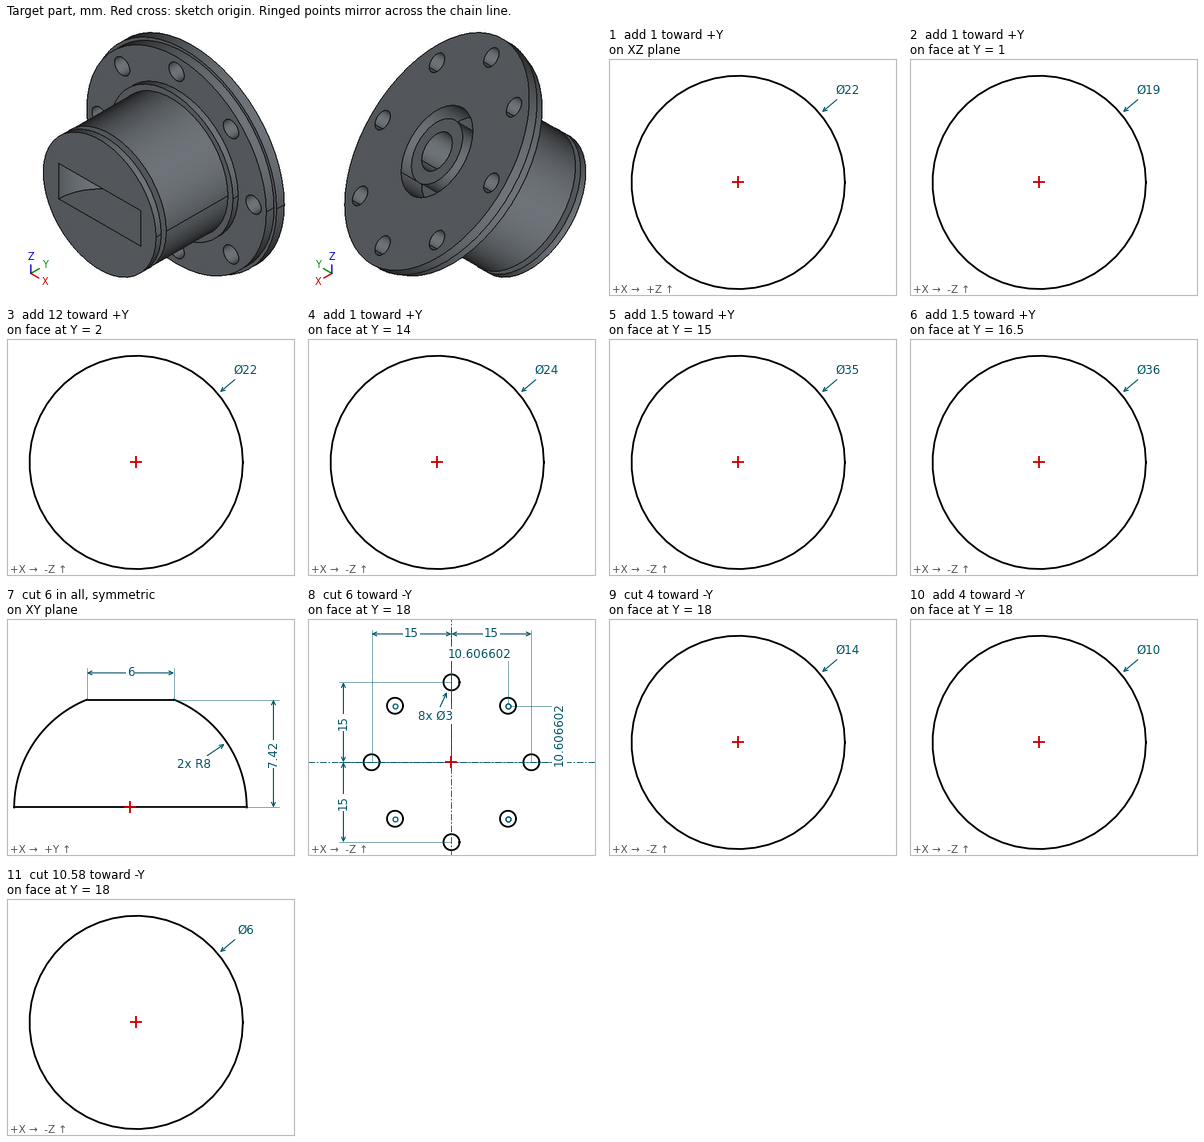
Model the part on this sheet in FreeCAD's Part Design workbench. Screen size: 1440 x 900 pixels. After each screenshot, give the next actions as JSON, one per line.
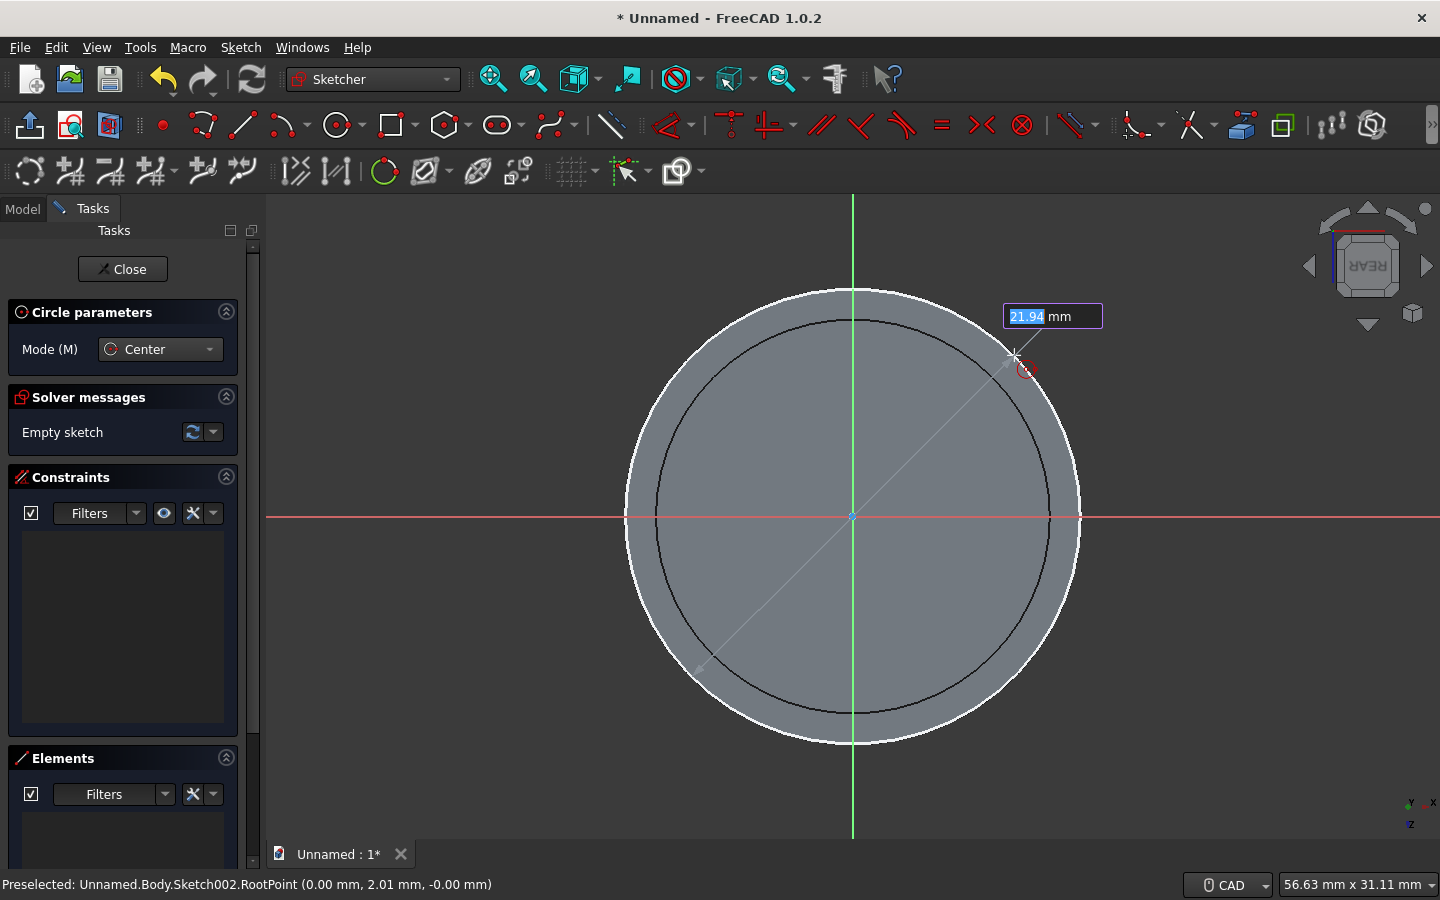
{"action": "type", "text": "22"}
{"action": "key", "text": "Return"}
{"action": "key", "text": "Escape"}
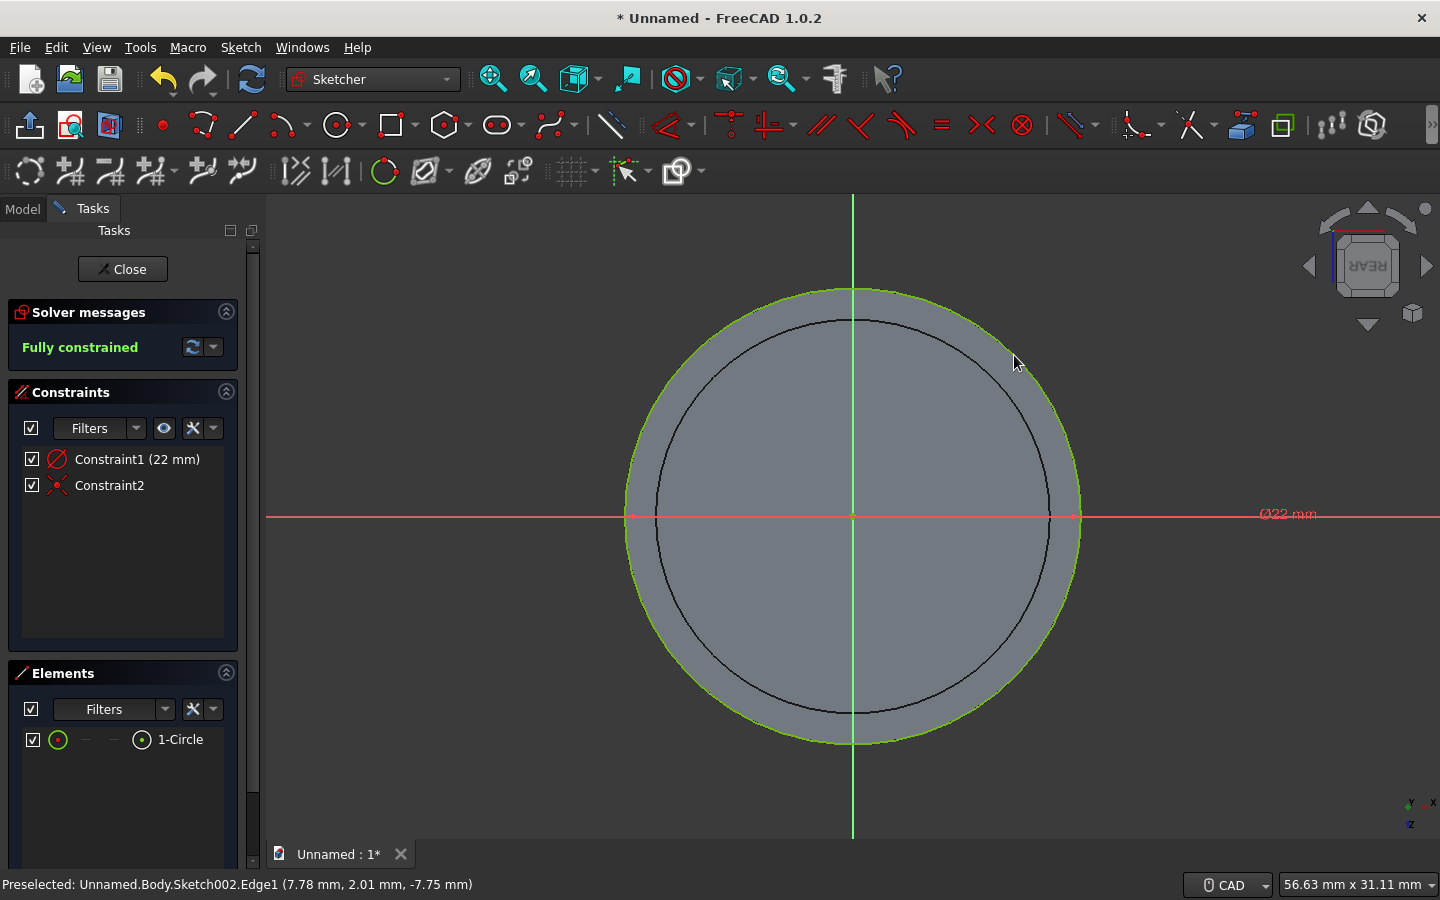
{"action": "left_click", "coordinate": [123, 269]}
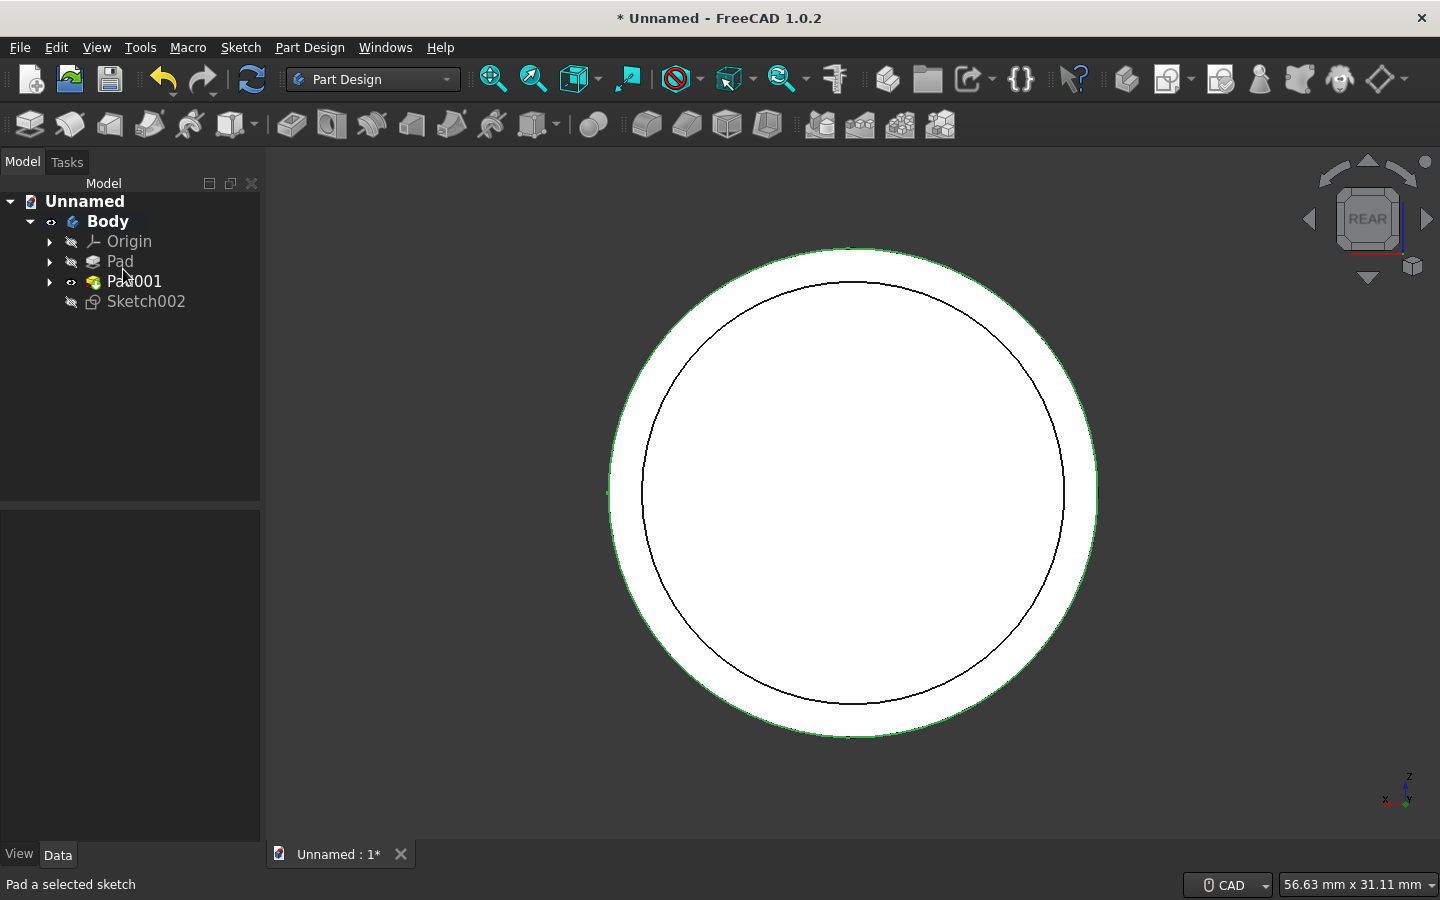
{"action": "left_click", "coordinate": [30, 124]}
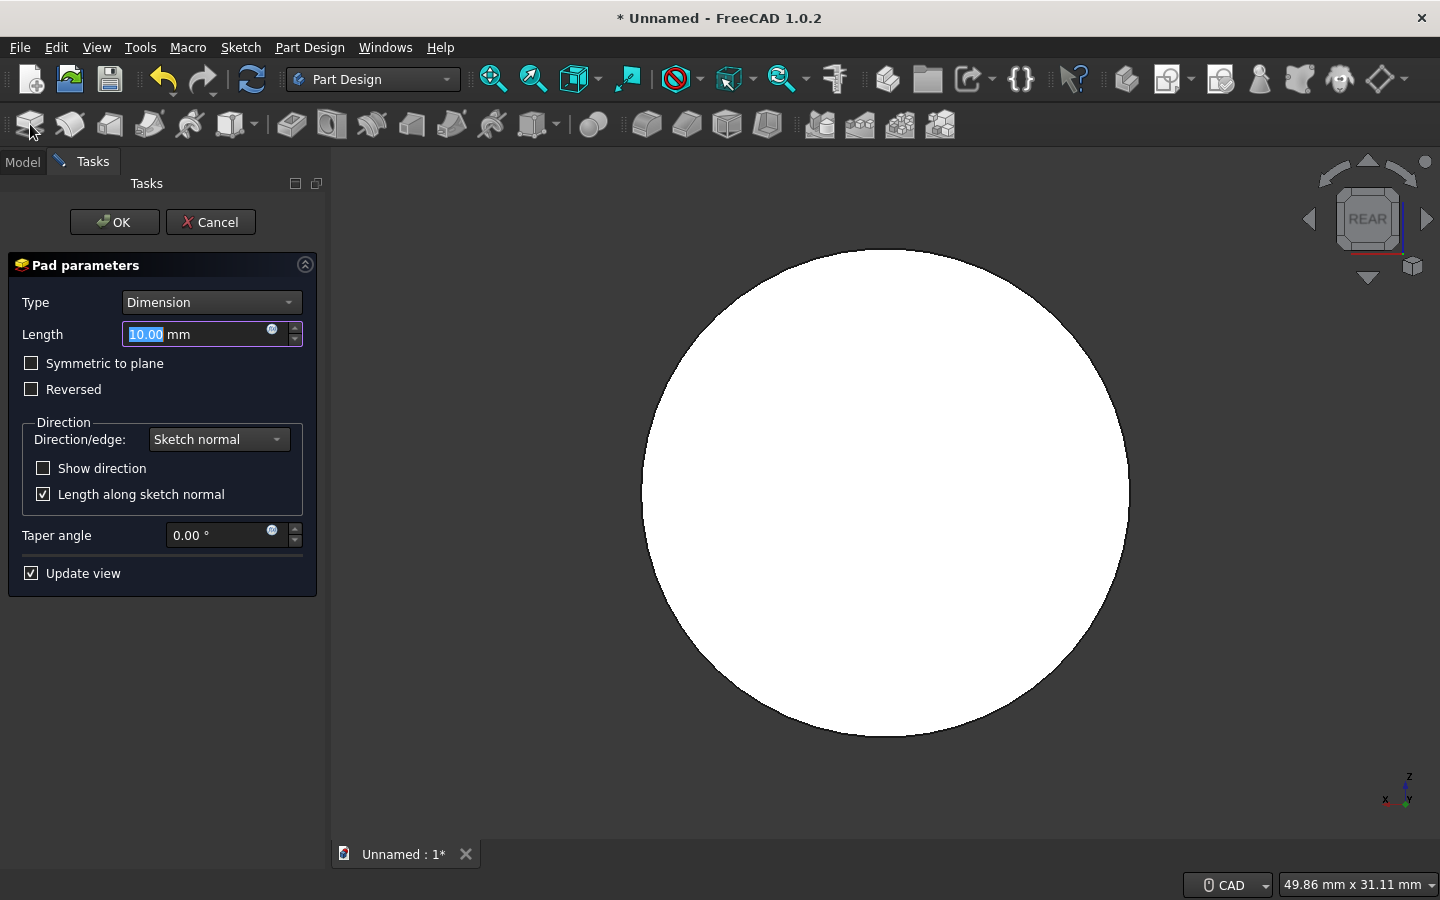
{"action": "type", "text": "12"}
{"action": "key", "text": "Tab"}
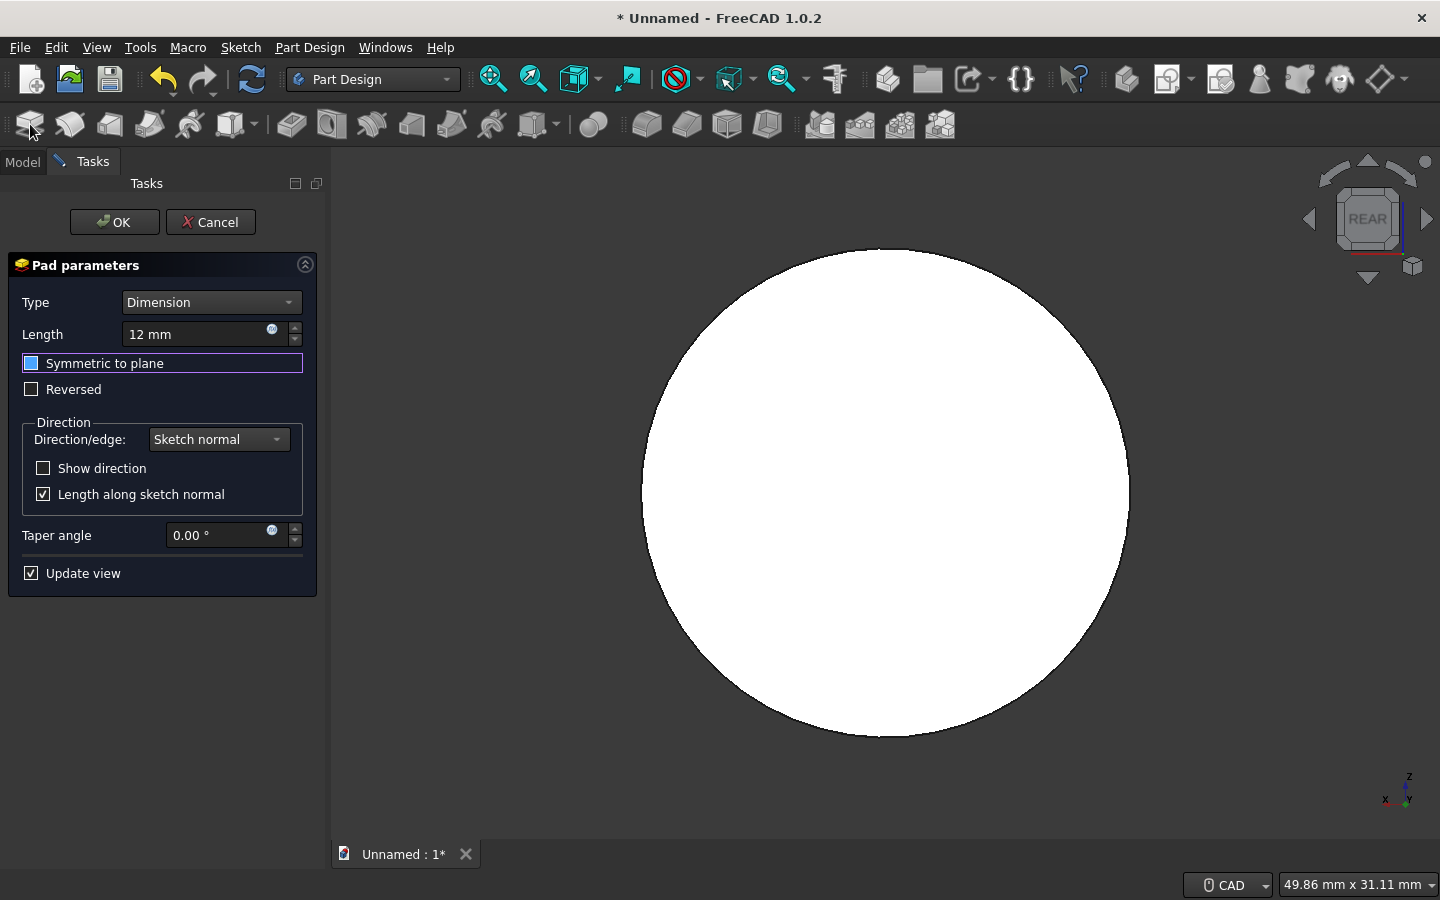
{"action": "left_click", "coordinate": [115, 222]}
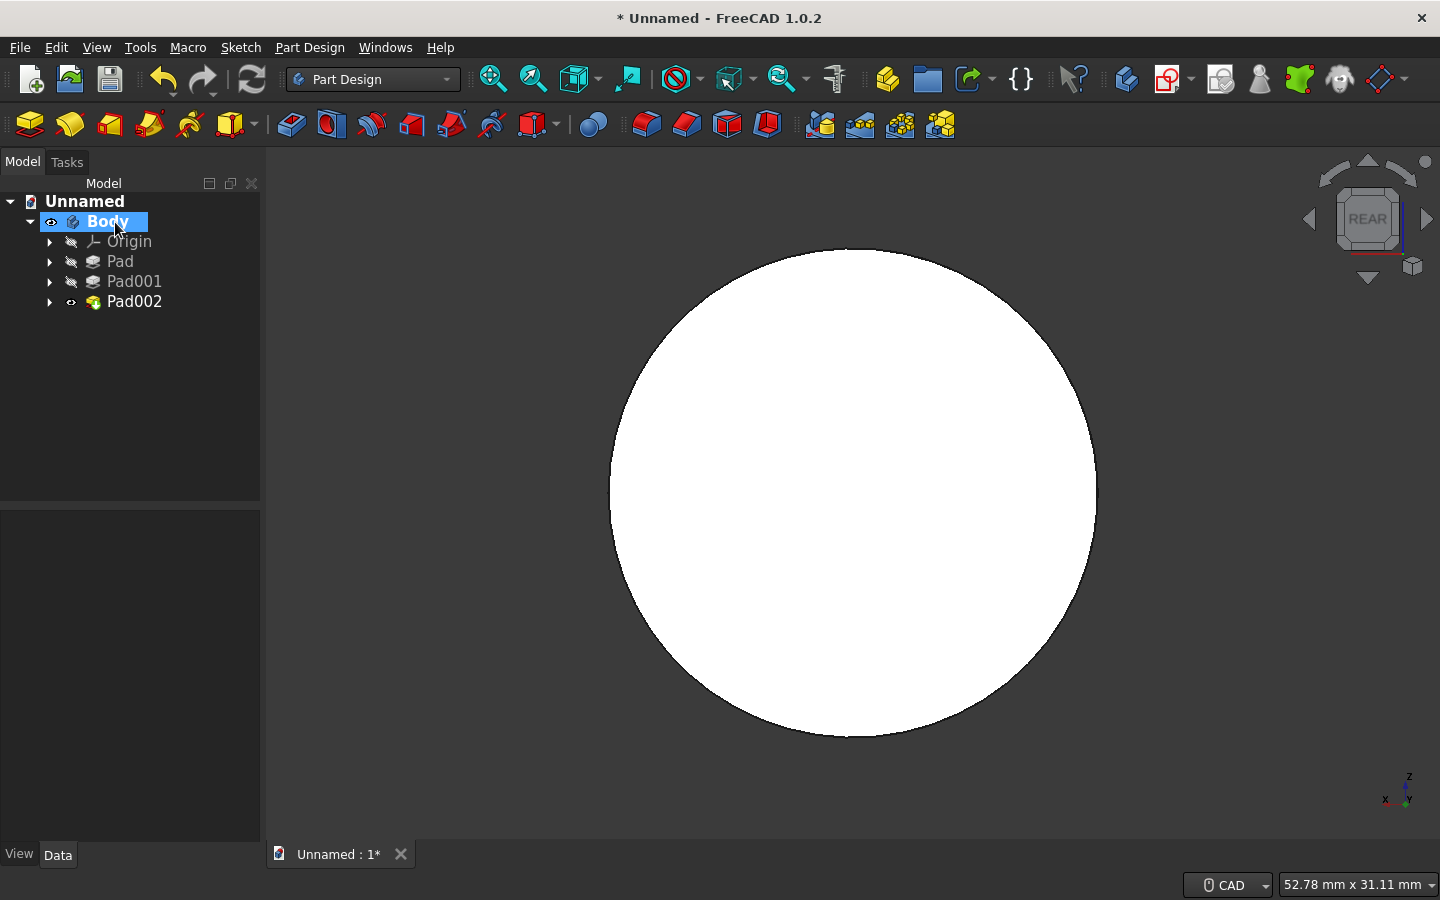
{"action": "left_click", "coordinate": [853, 492]}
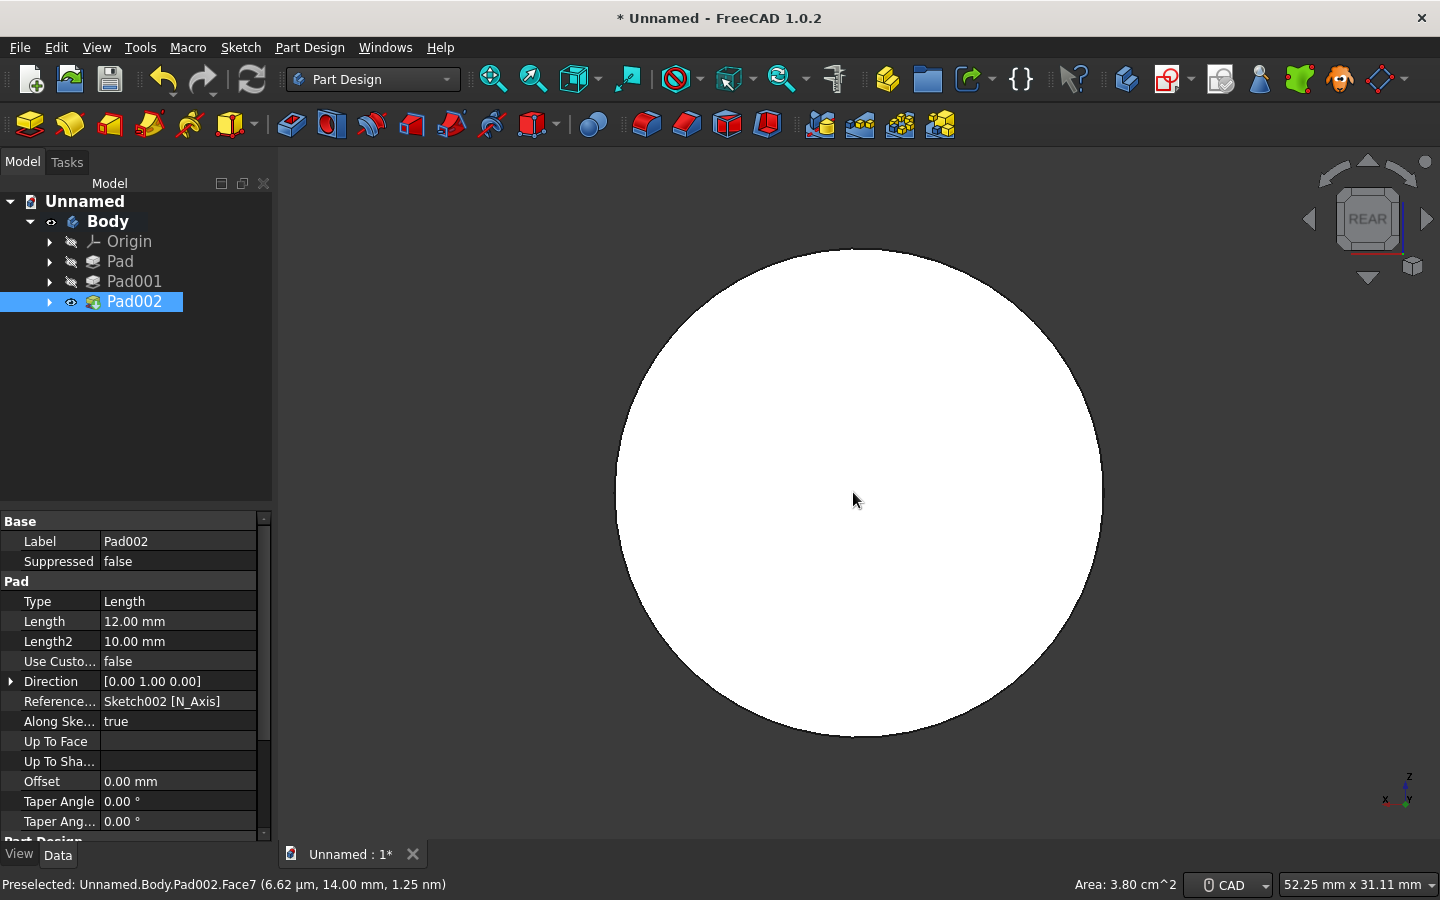
{"action": "left_click", "coordinate": [1168, 80]}